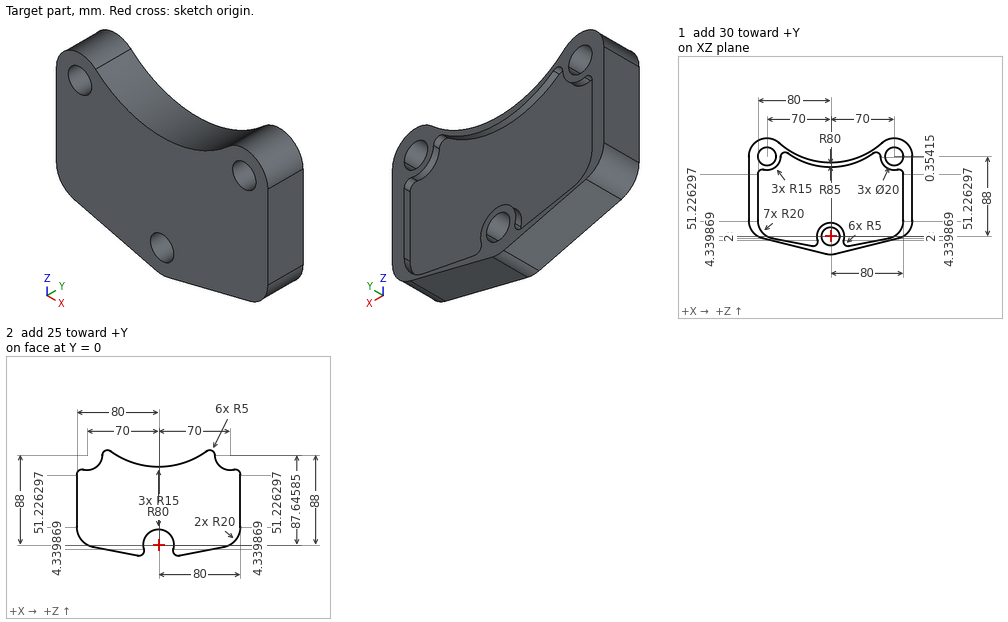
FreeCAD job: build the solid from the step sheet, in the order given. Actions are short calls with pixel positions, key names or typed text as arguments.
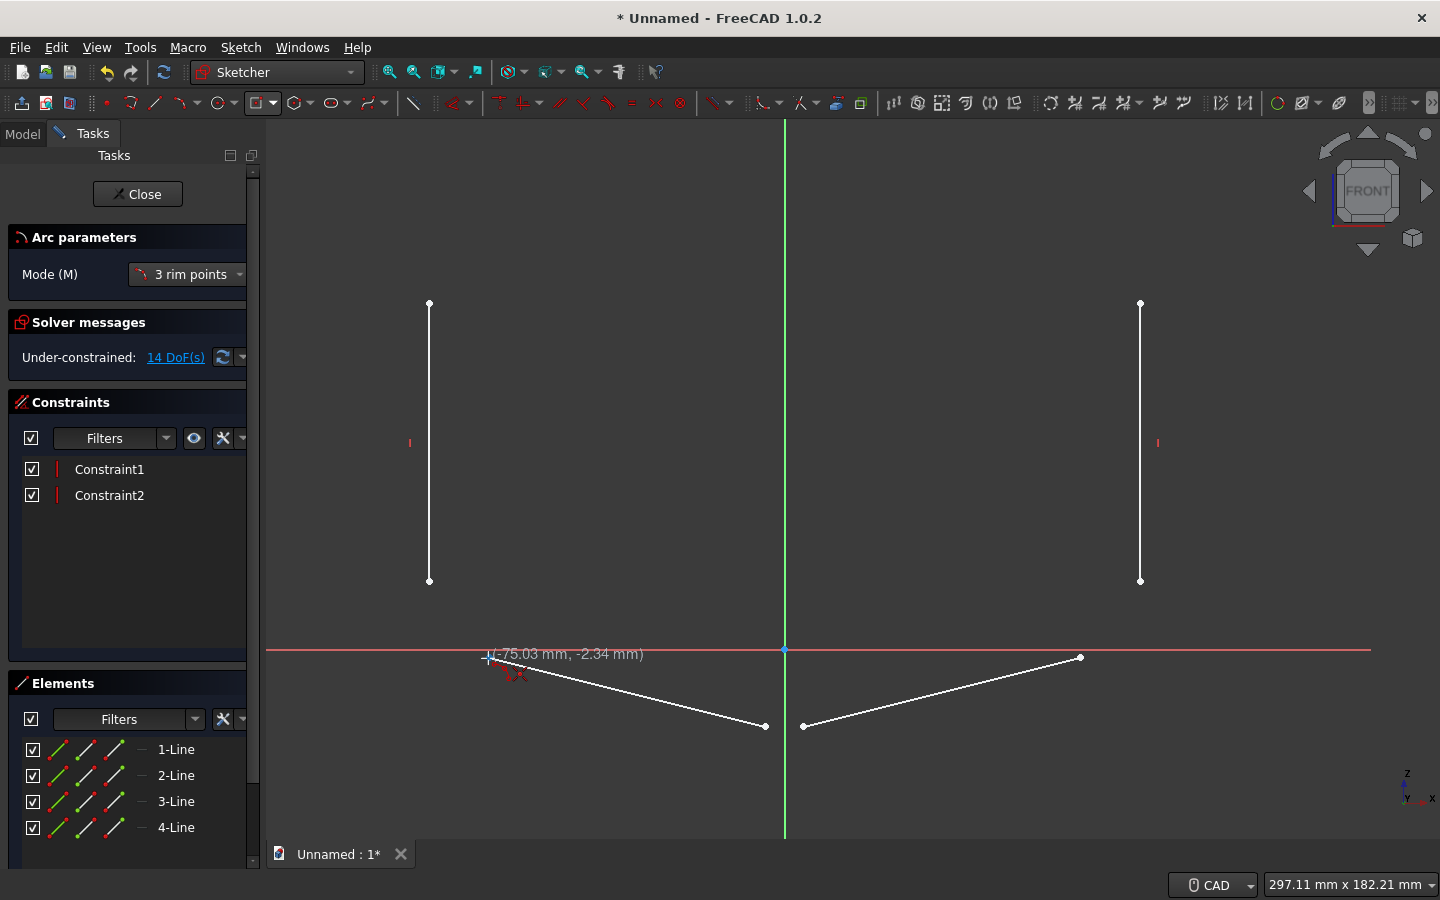
click(429, 303)
click(561, 243)
click(476, 230)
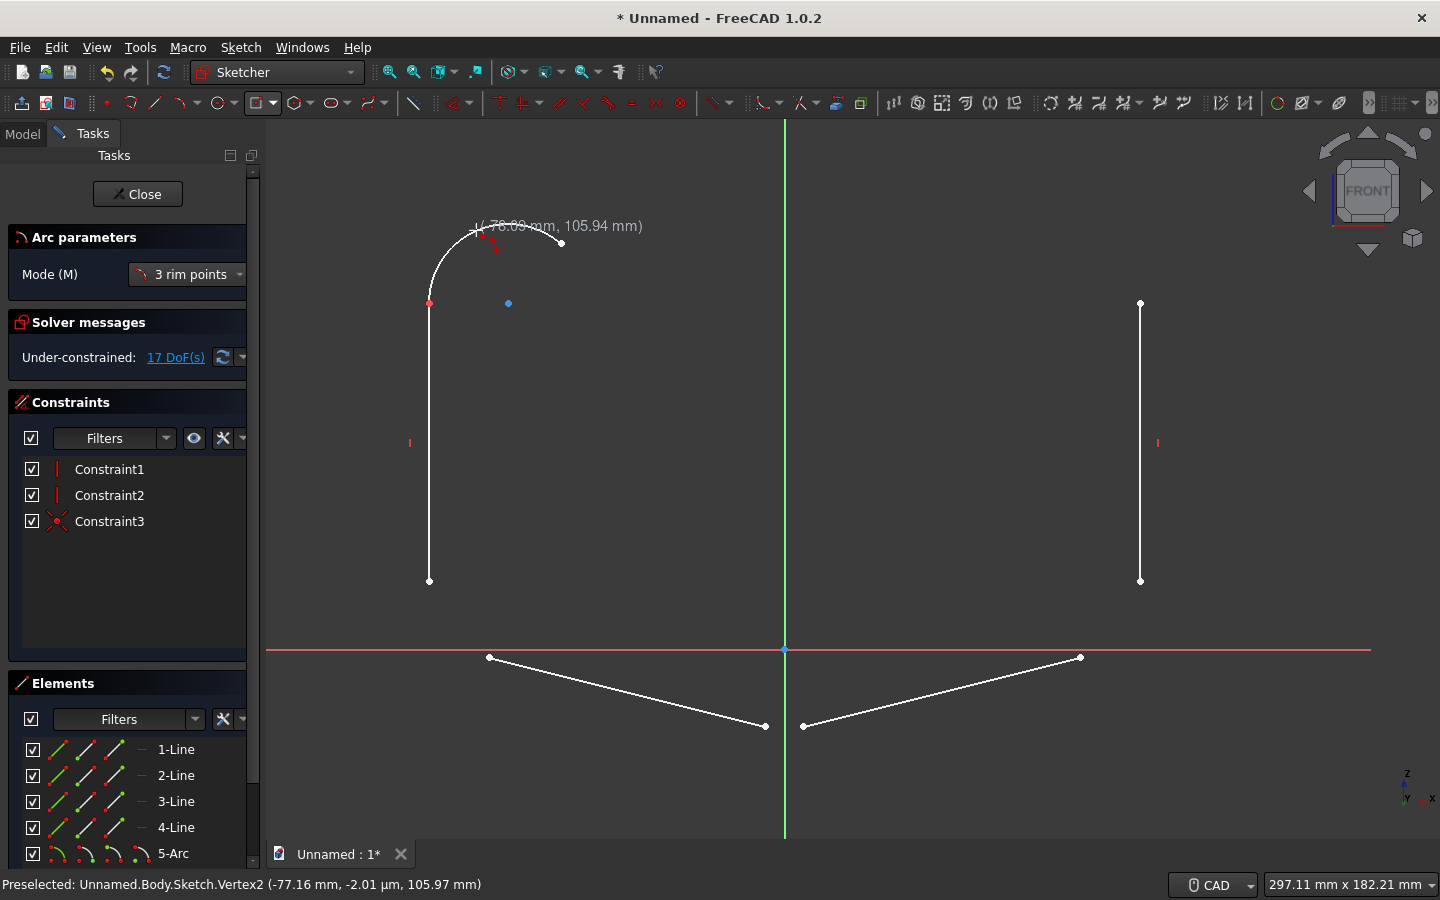
click(561, 244)
click(1009, 243)
click(736, 325)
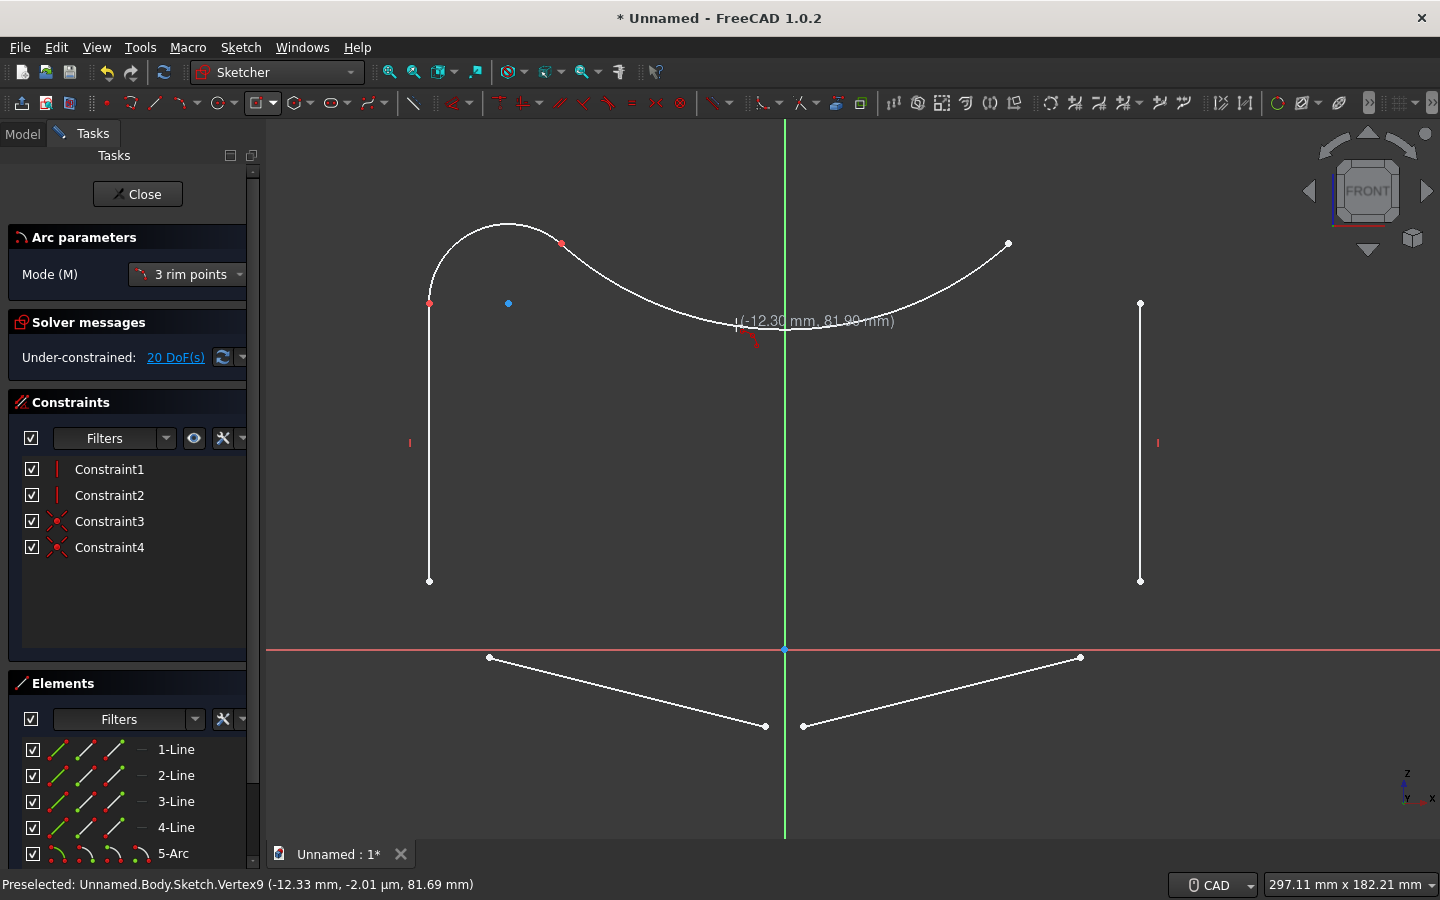
click(1009, 244)
click(1140, 303)
click(1093, 230)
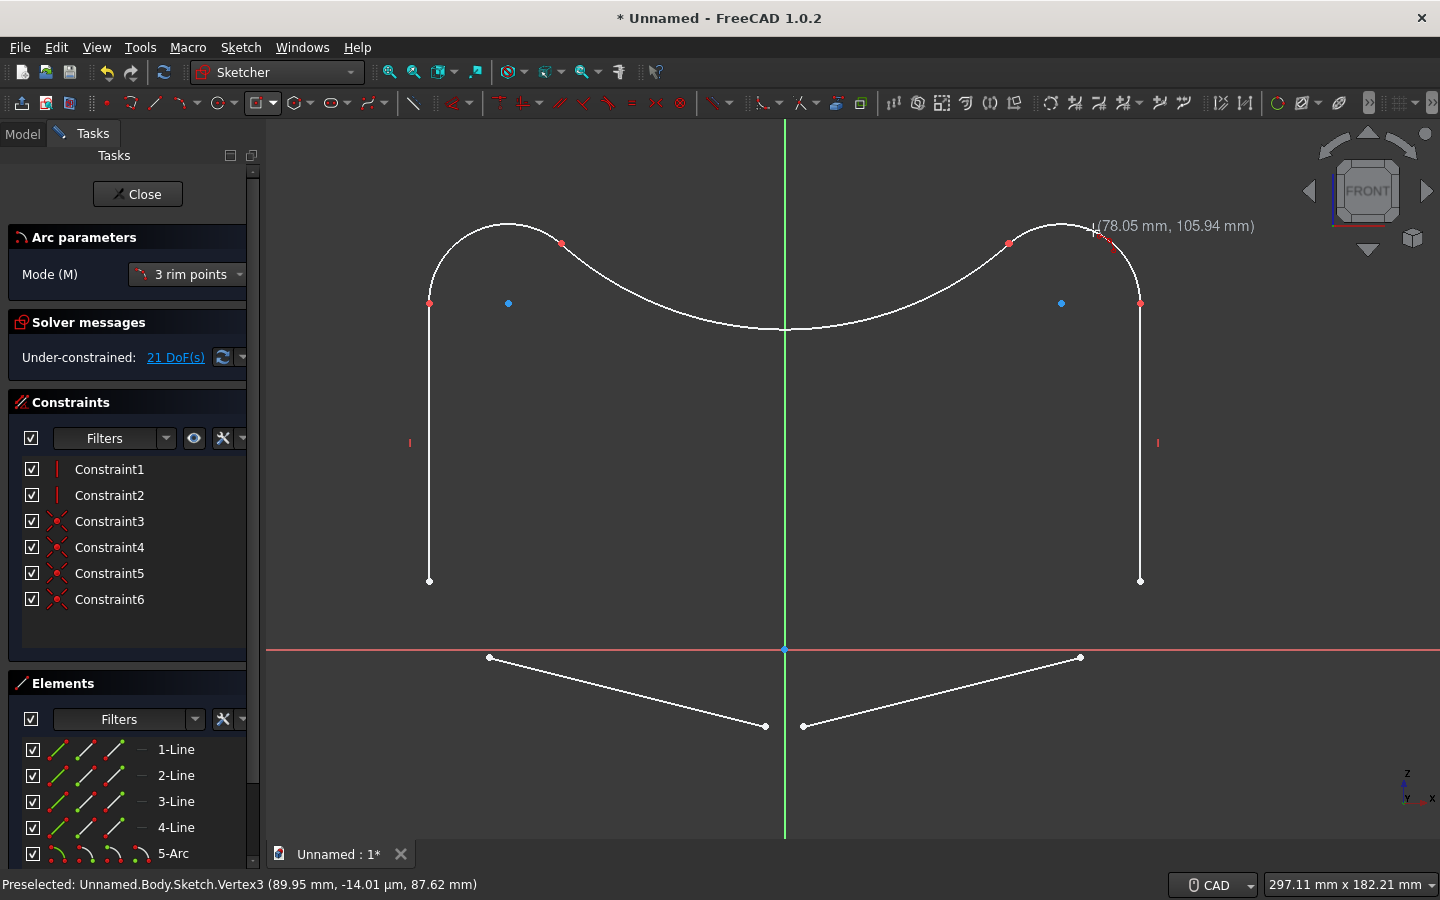
click(1140, 581)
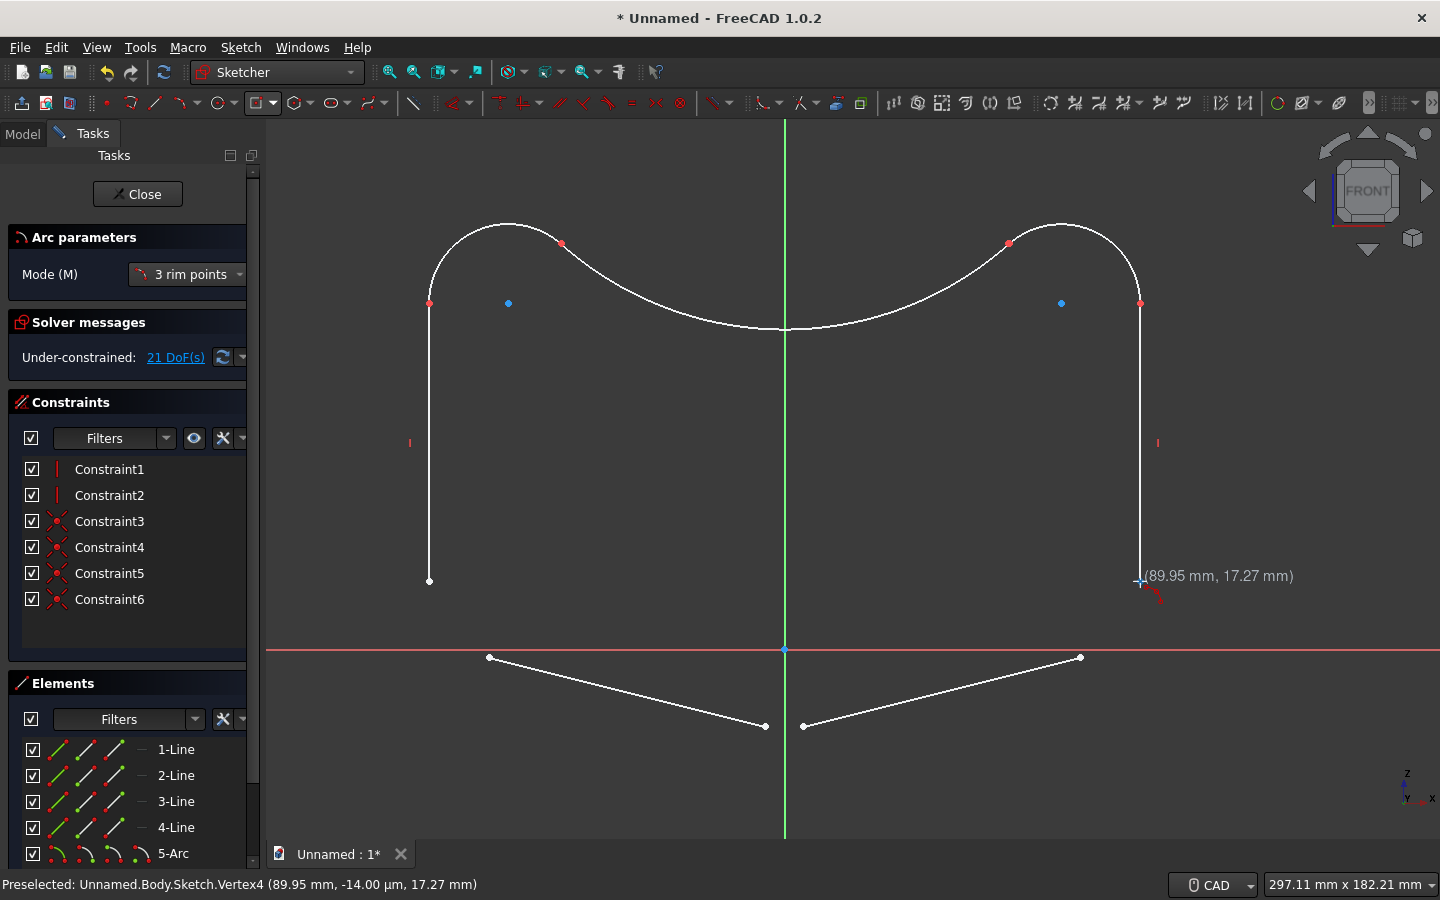
scroll(1080, 658, up, 4)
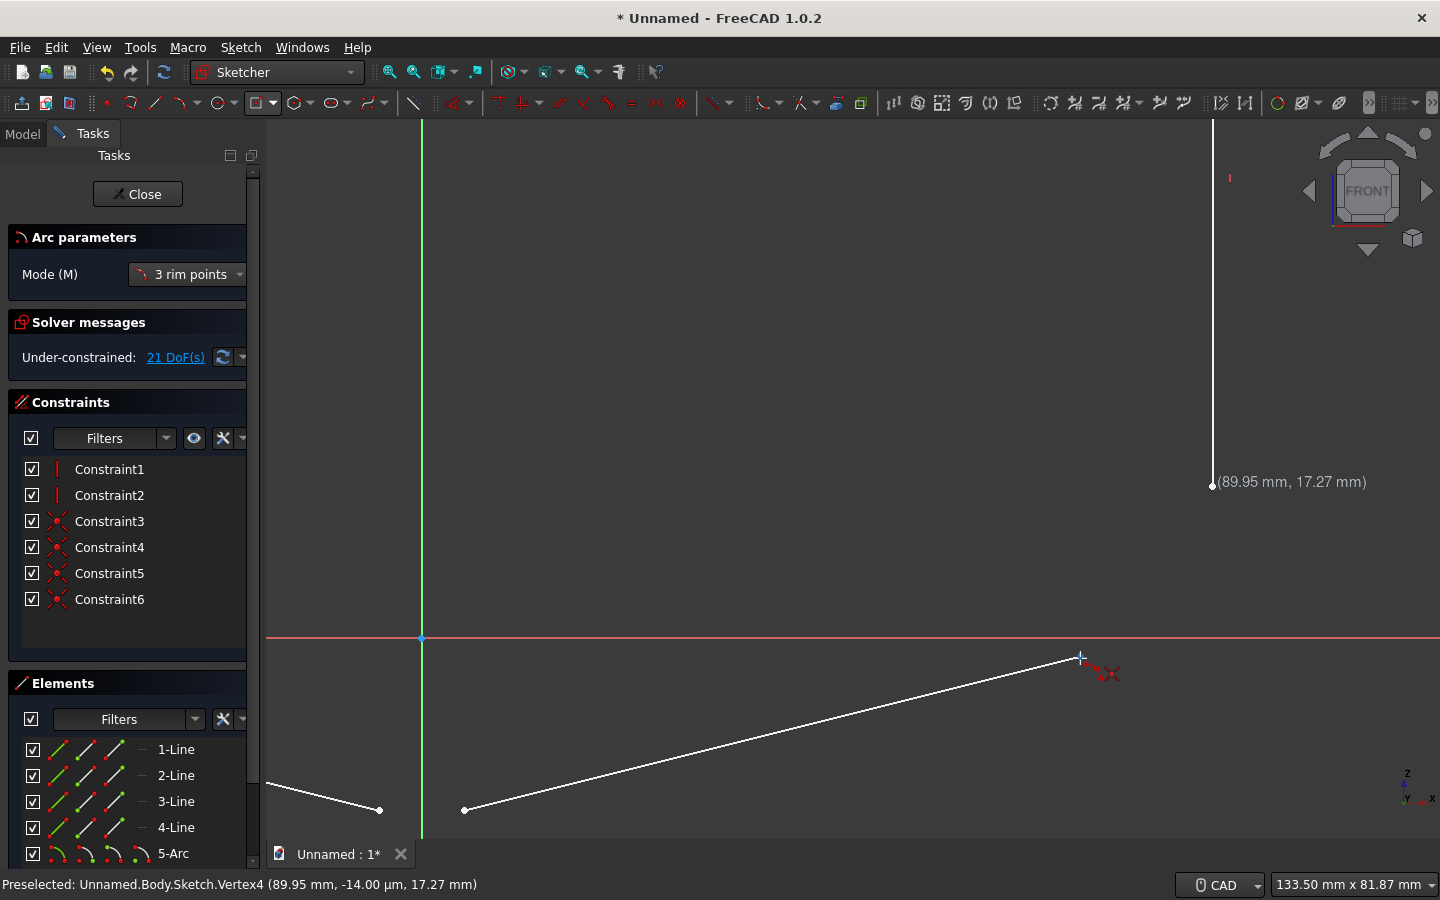
click(1080, 657)
click(1176, 594)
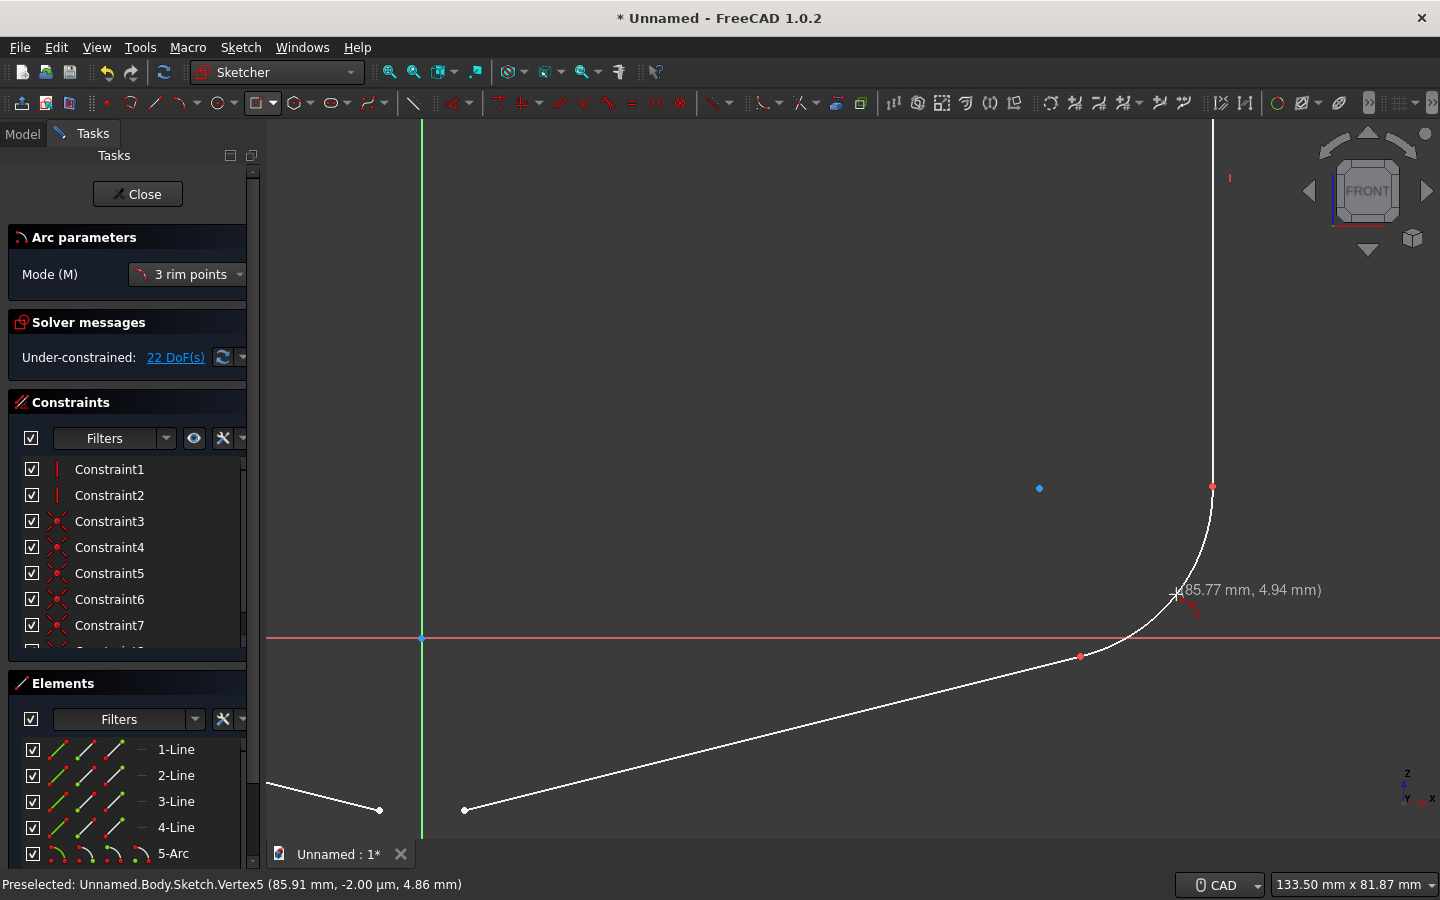
click(464, 811)
click(379, 811)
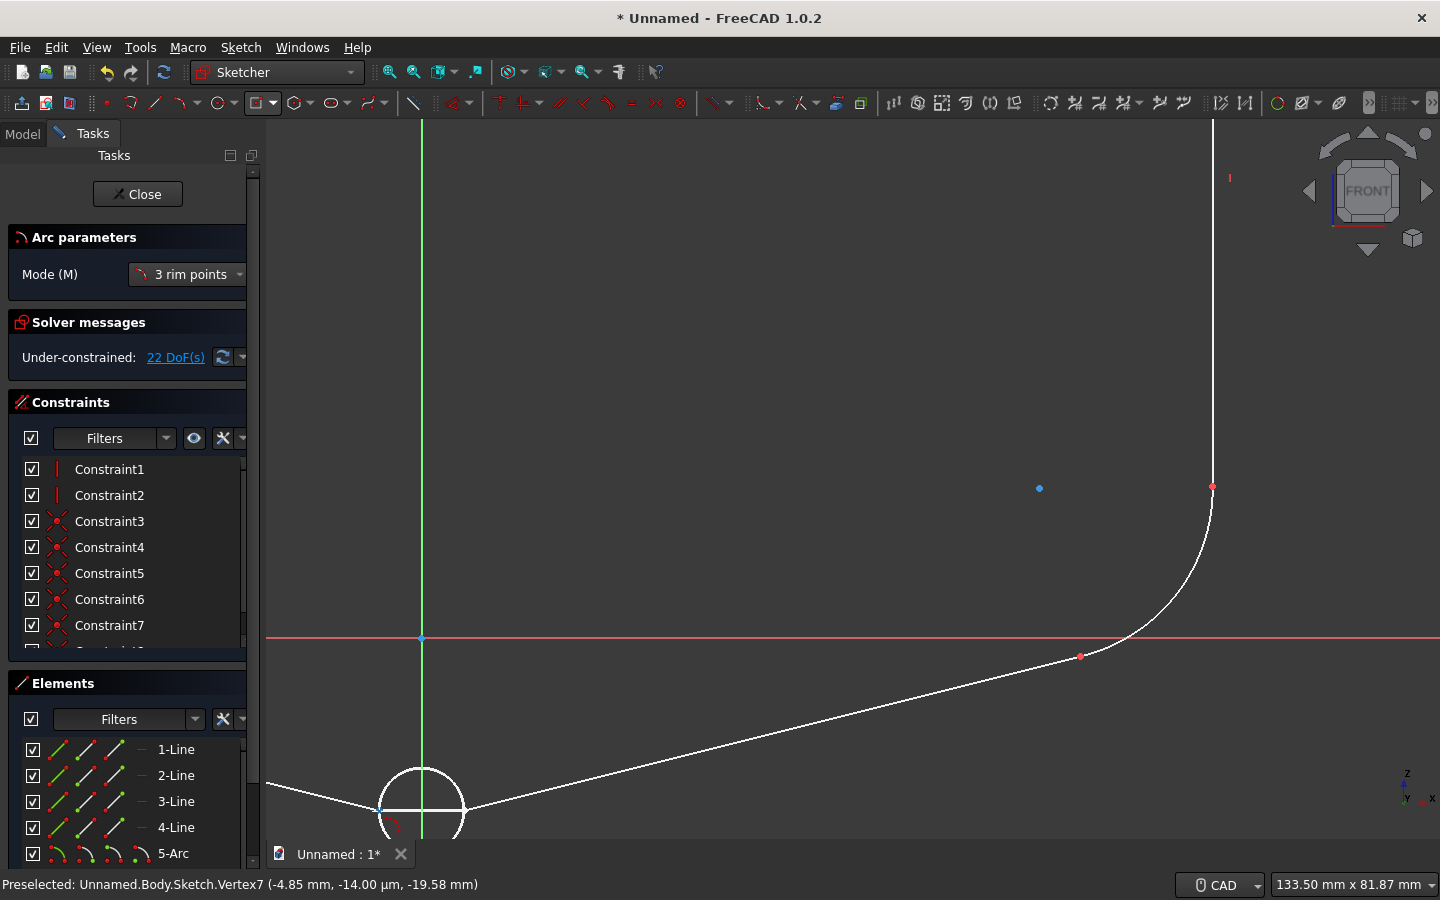
scroll(1081, 658, down, 4)